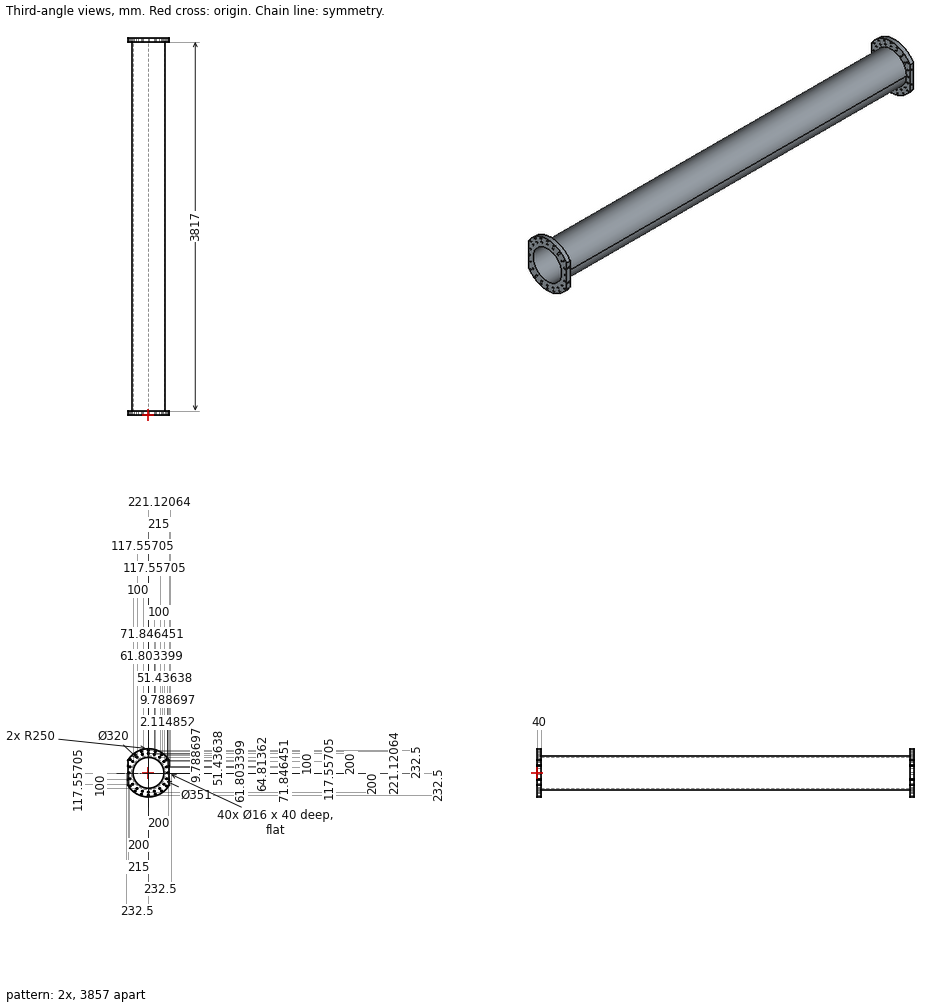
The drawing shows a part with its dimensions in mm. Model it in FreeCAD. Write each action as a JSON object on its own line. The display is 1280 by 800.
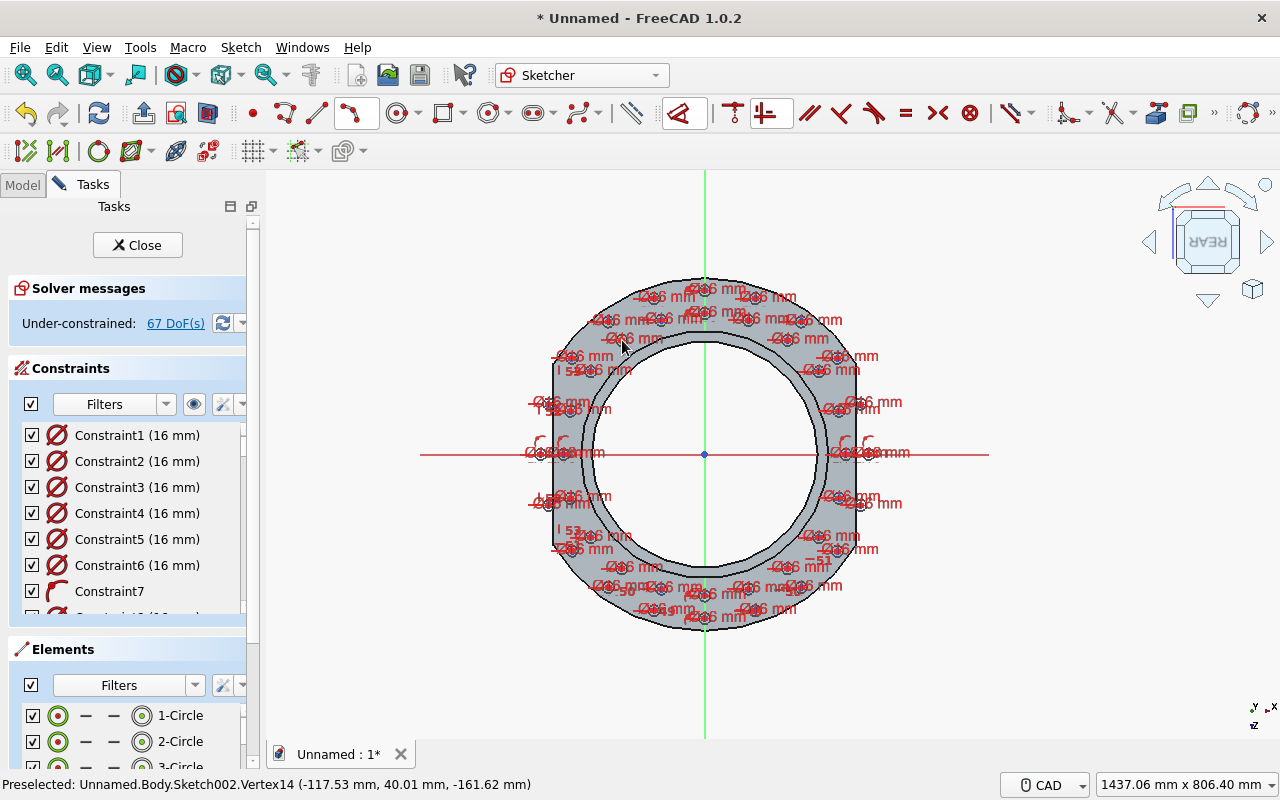
{"action": "left_click", "coordinate": [788, 114]}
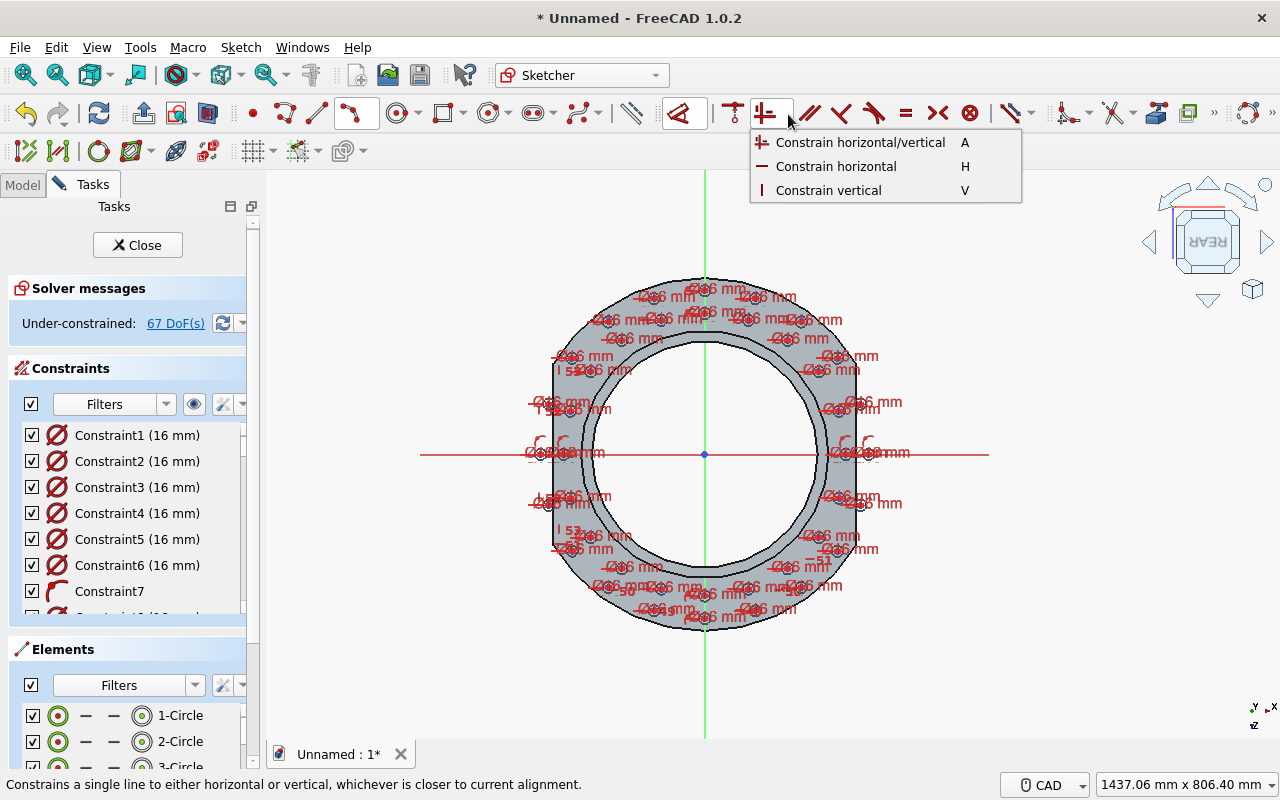
{"action": "left_click", "coordinate": [886, 190]}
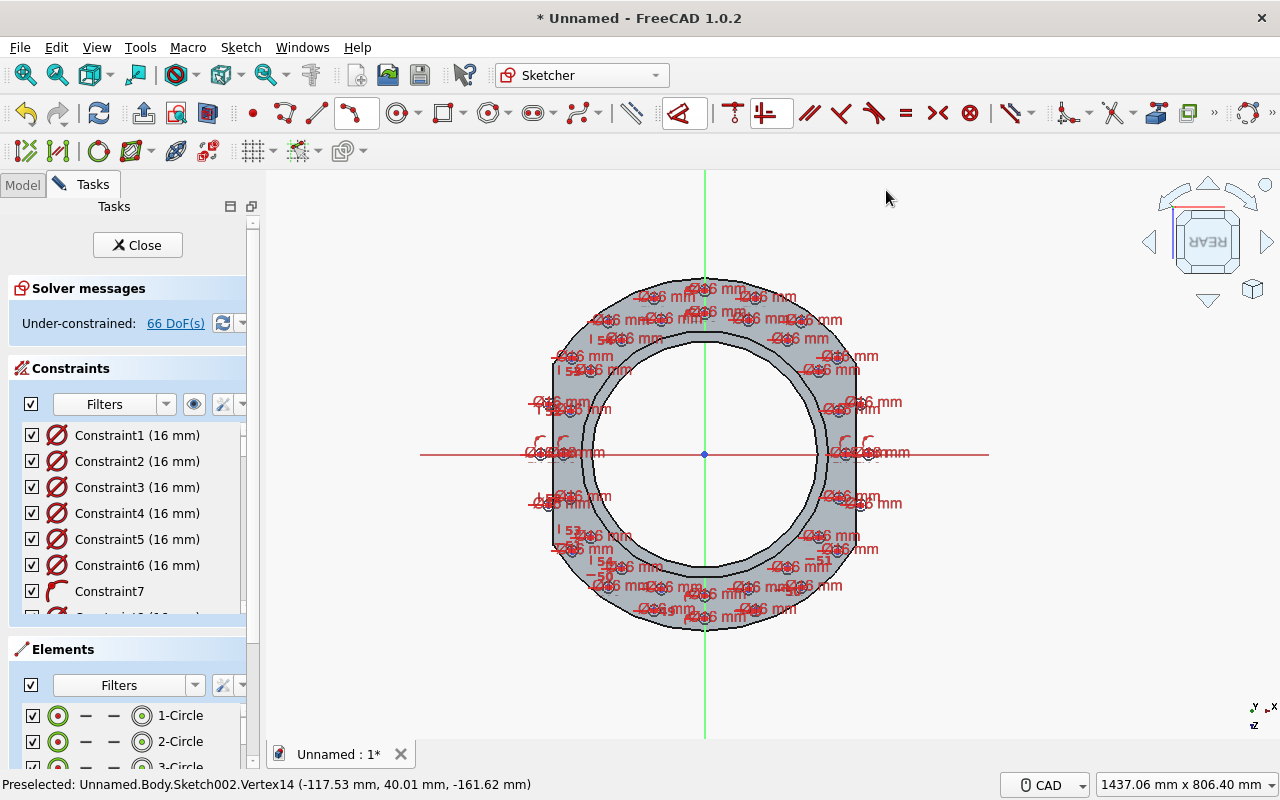
{"action": "left_click", "coordinate": [661, 320]}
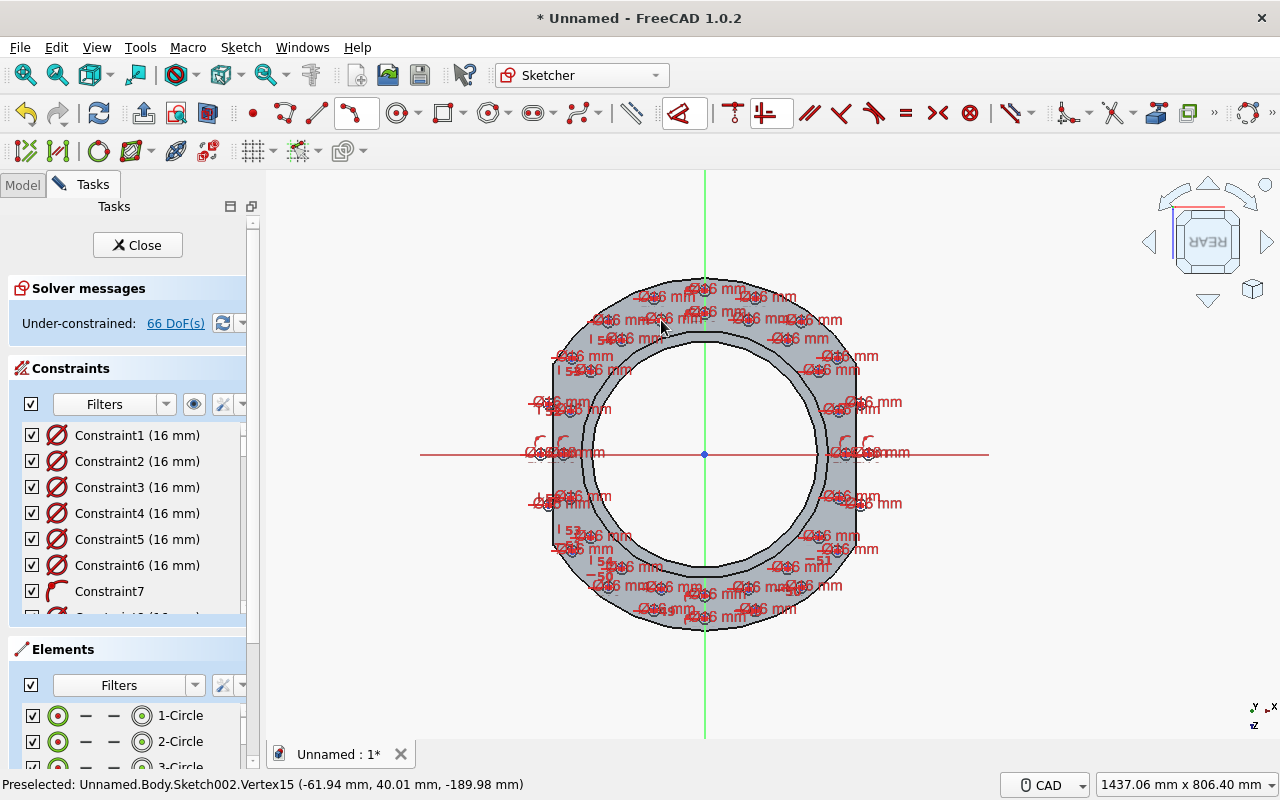
{"action": "left_click", "coordinate": [748, 320]}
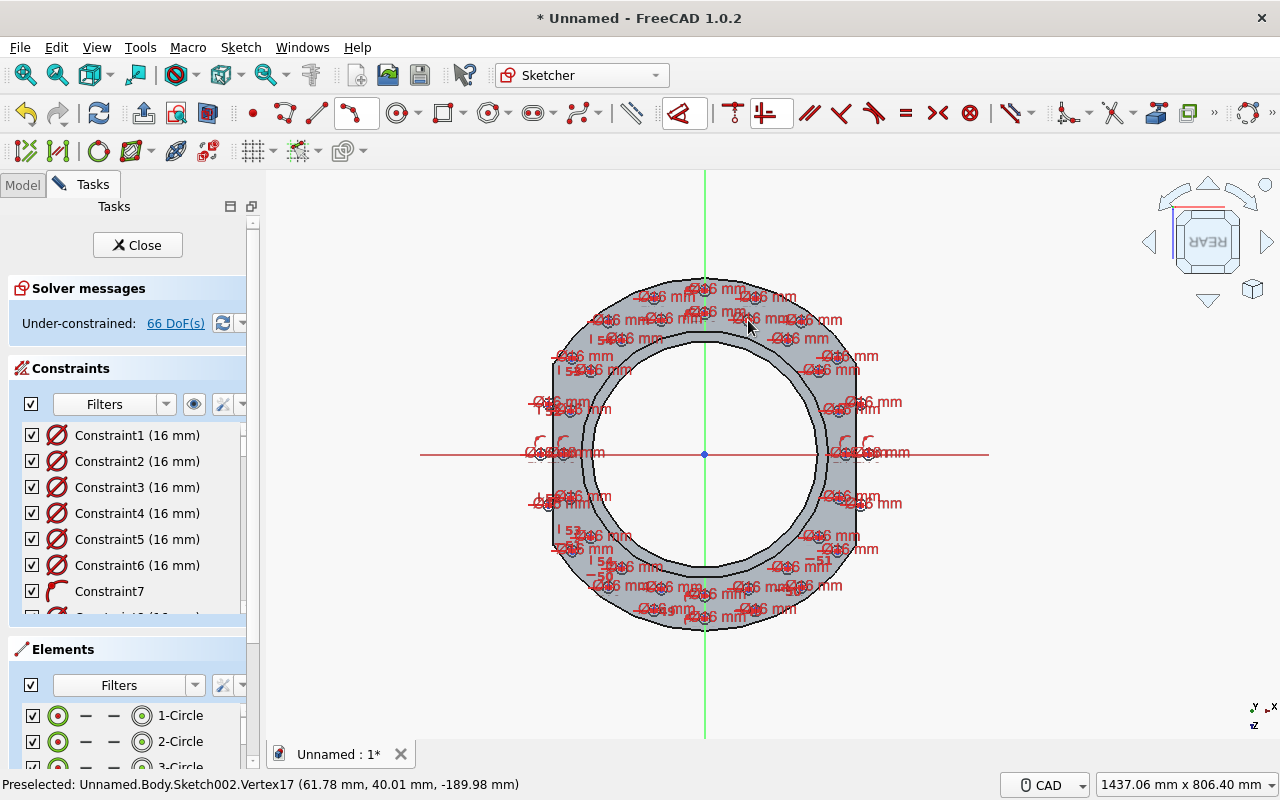
{"action": "left_click", "coordinate": [788, 114]}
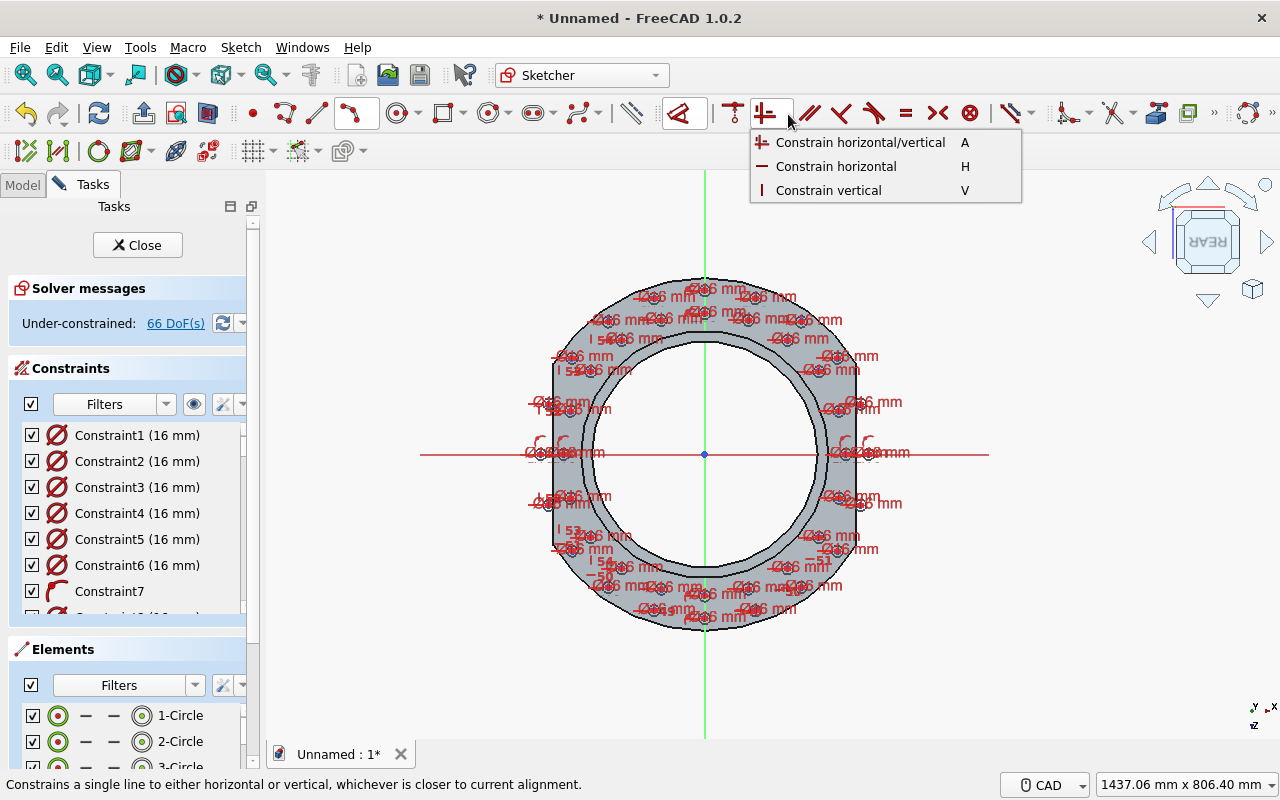
{"action": "left_click", "coordinate": [886, 166]}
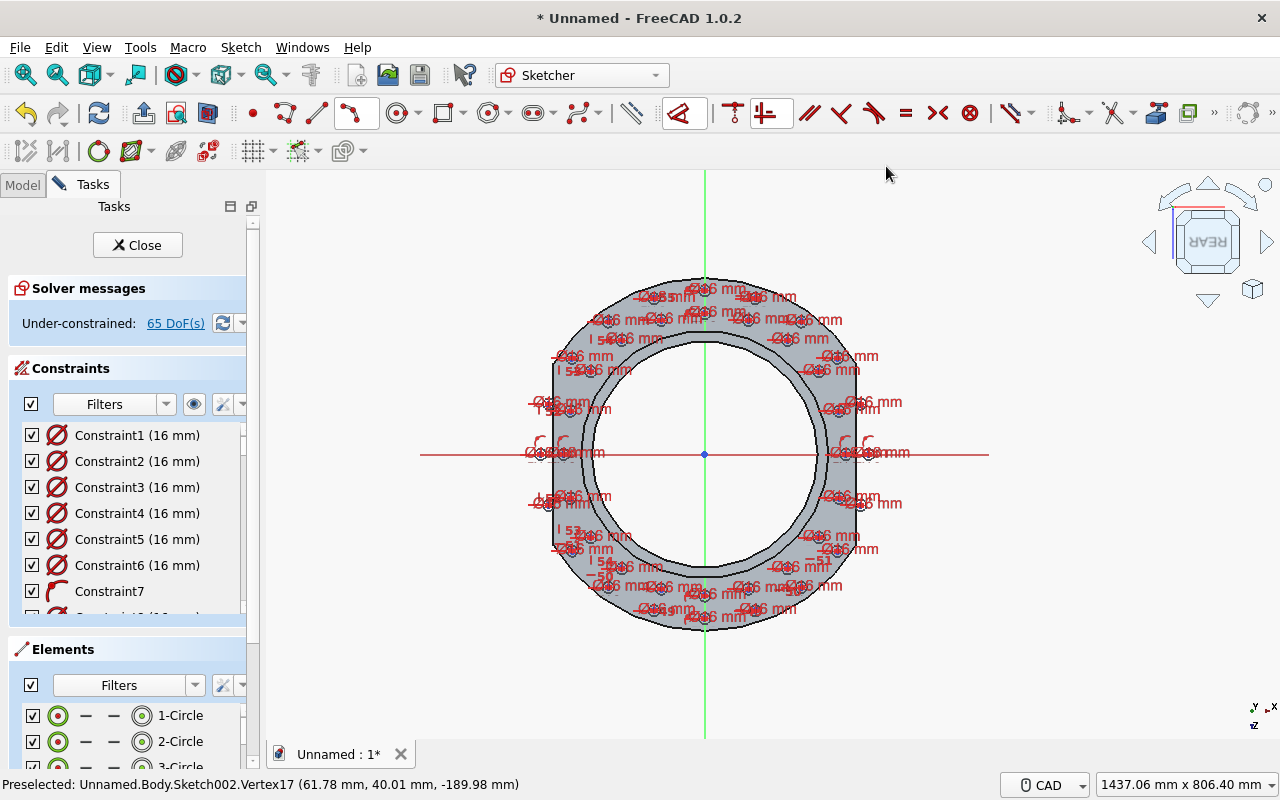
{"action": "left_click", "coordinate": [622, 340]}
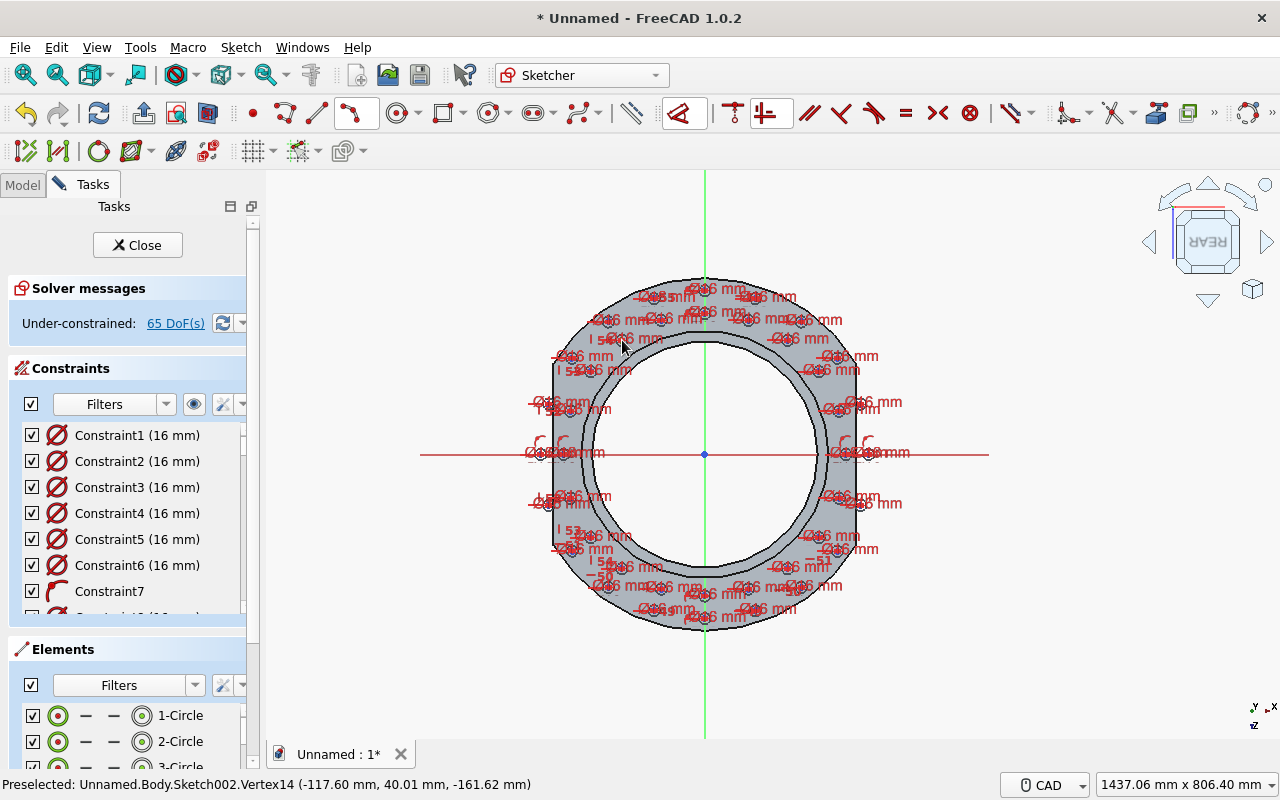
{"action": "left_click", "coordinate": [788, 340]}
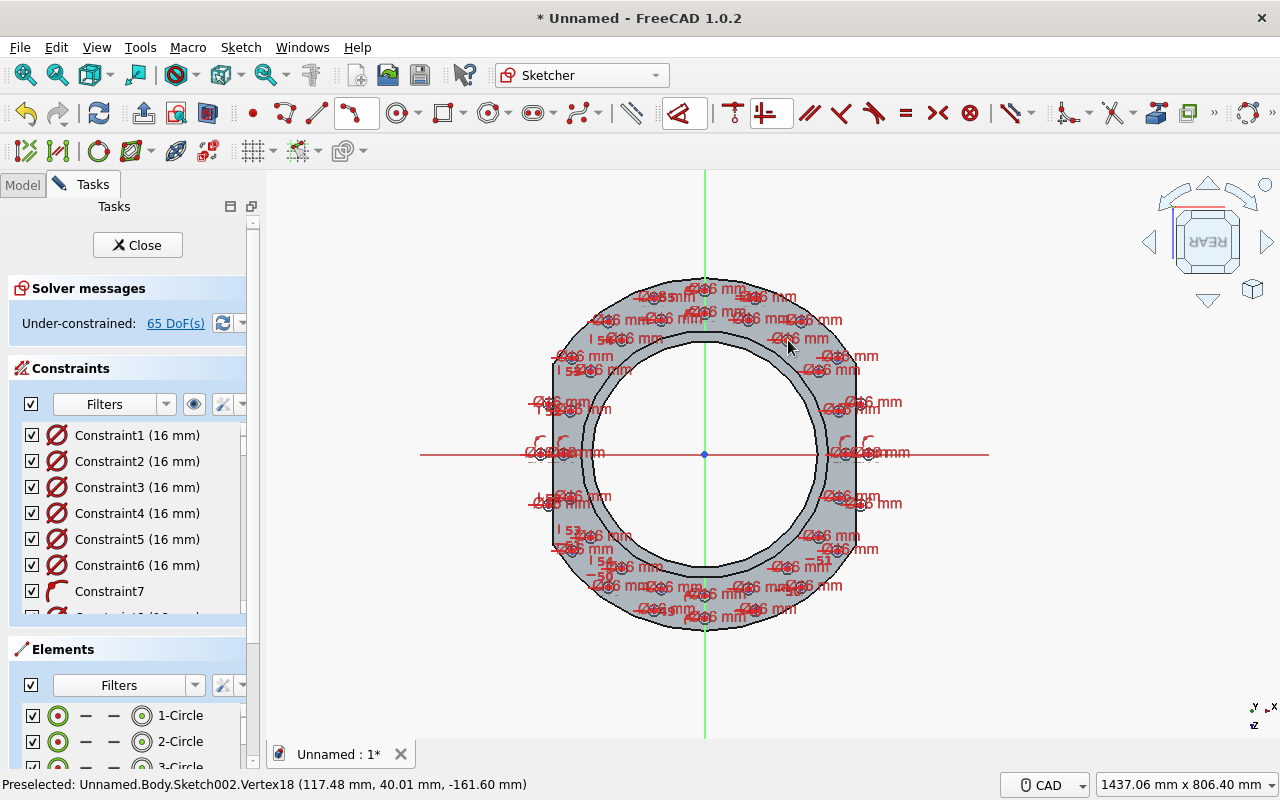
{"action": "key", "text": "h"}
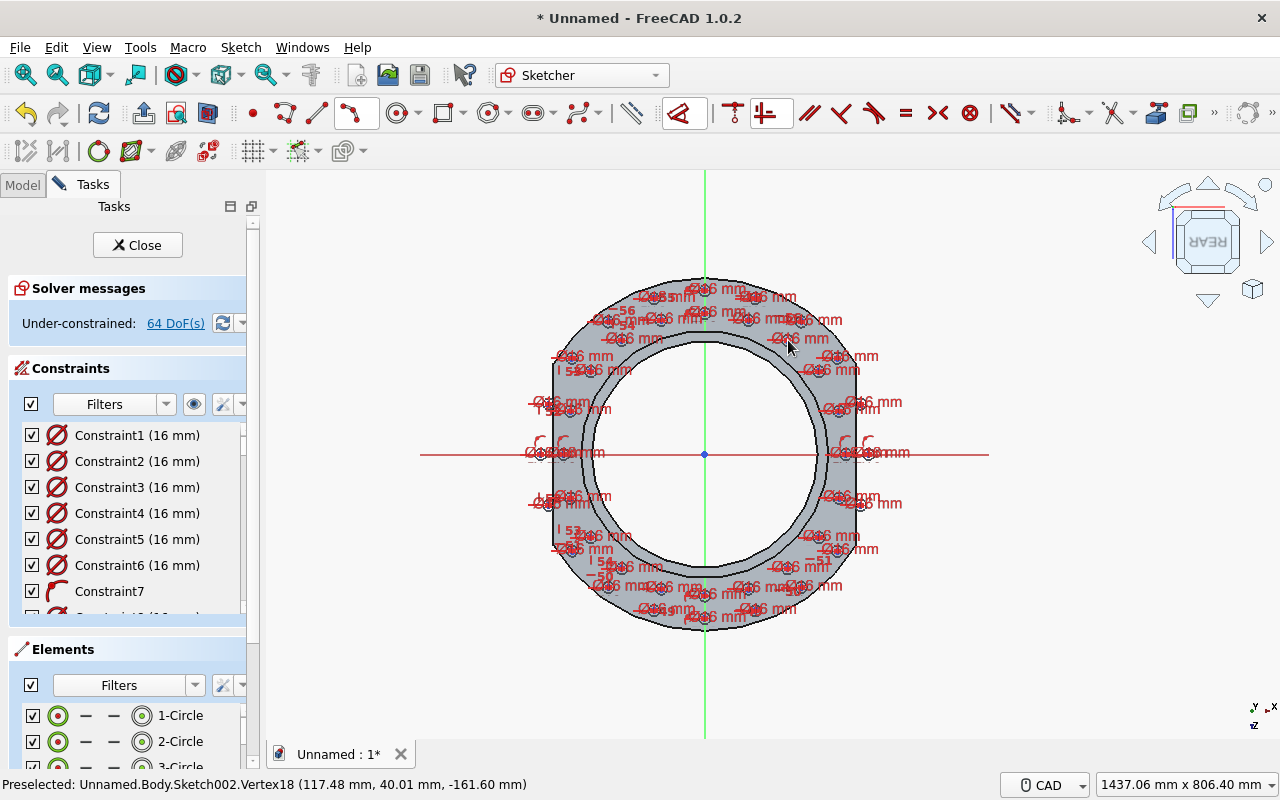
{"action": "left_click", "coordinate": [819, 538]}